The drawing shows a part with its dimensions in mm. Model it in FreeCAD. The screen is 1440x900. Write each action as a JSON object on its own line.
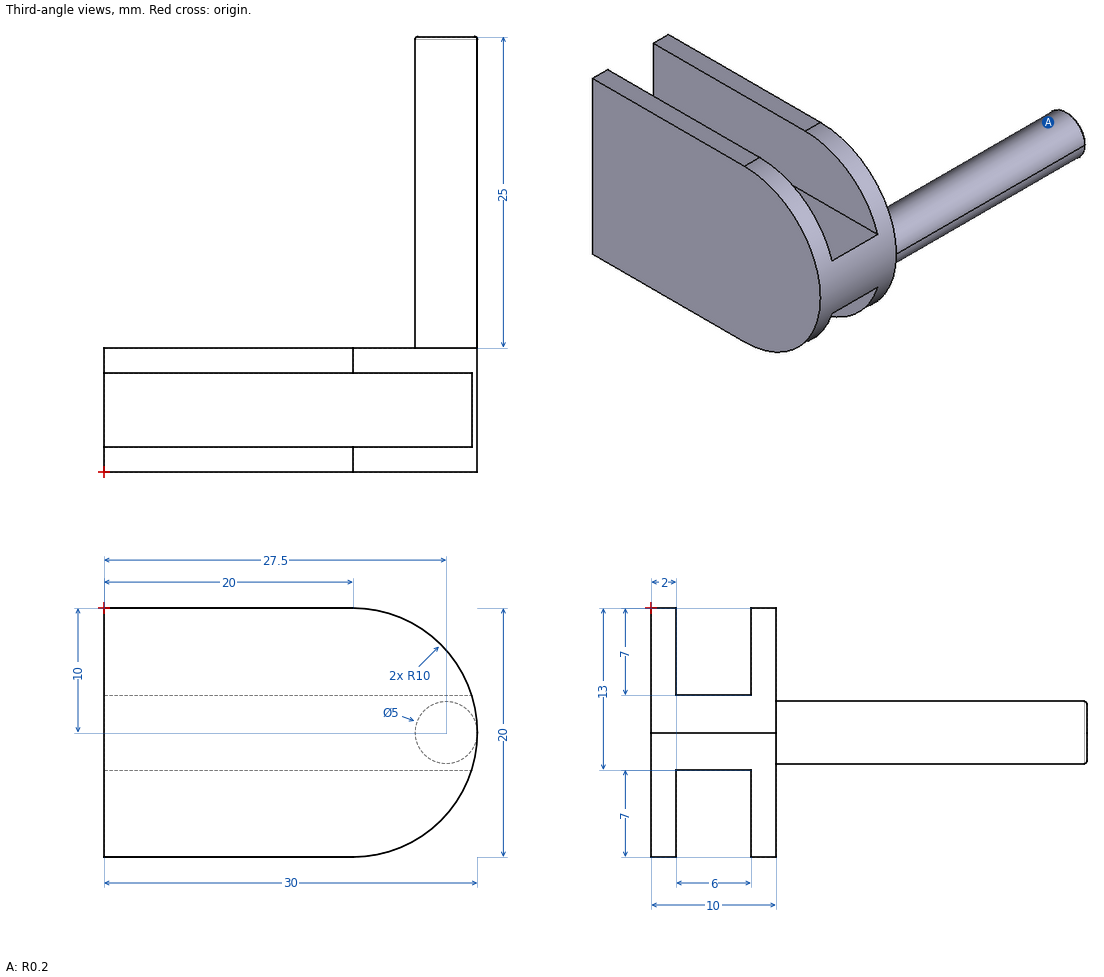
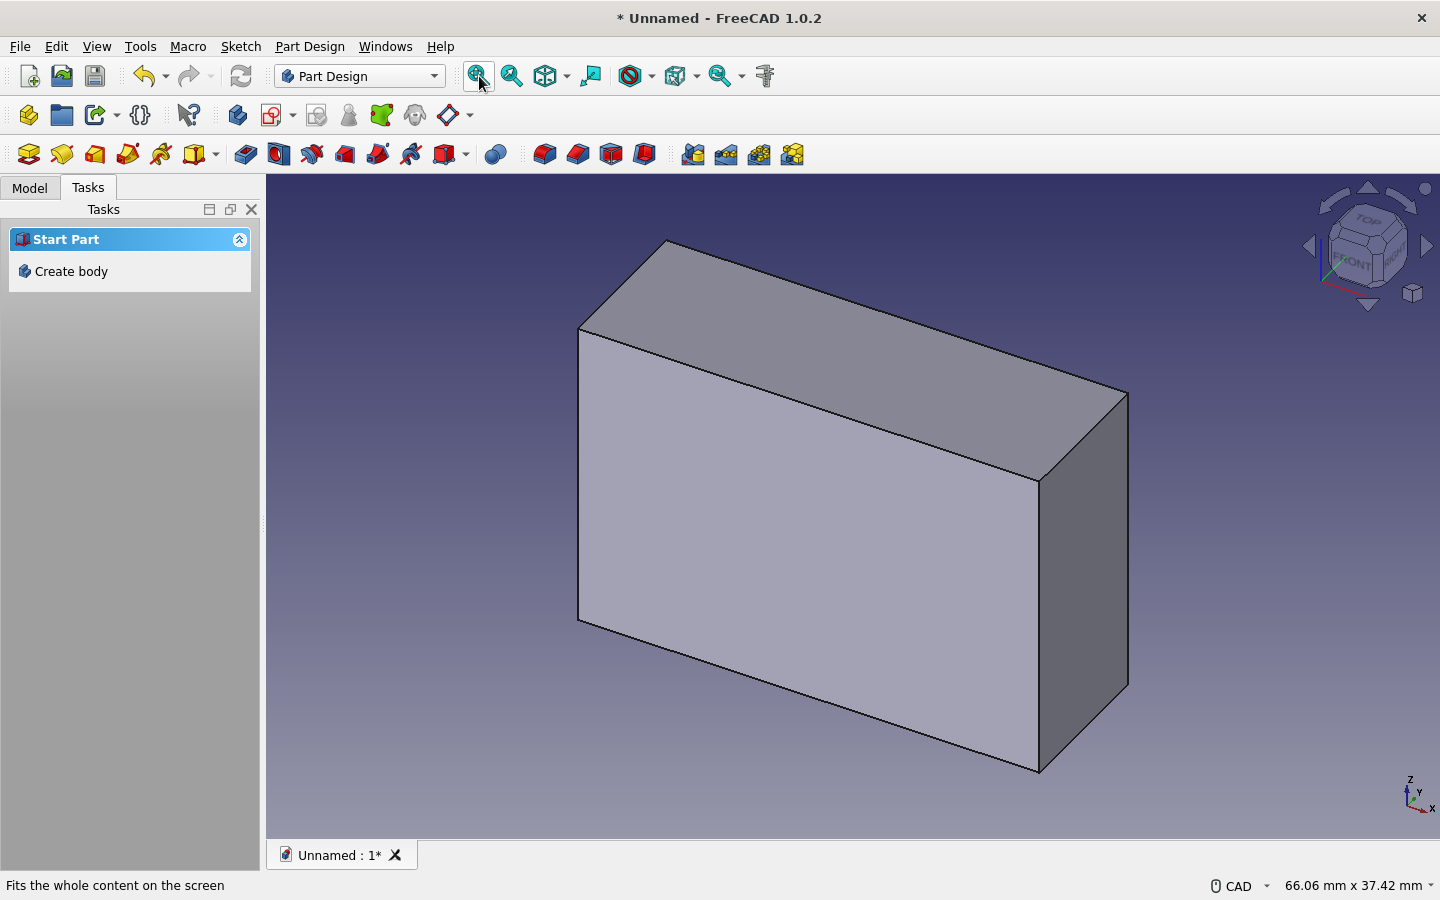
{"action": "key", "text": "6"}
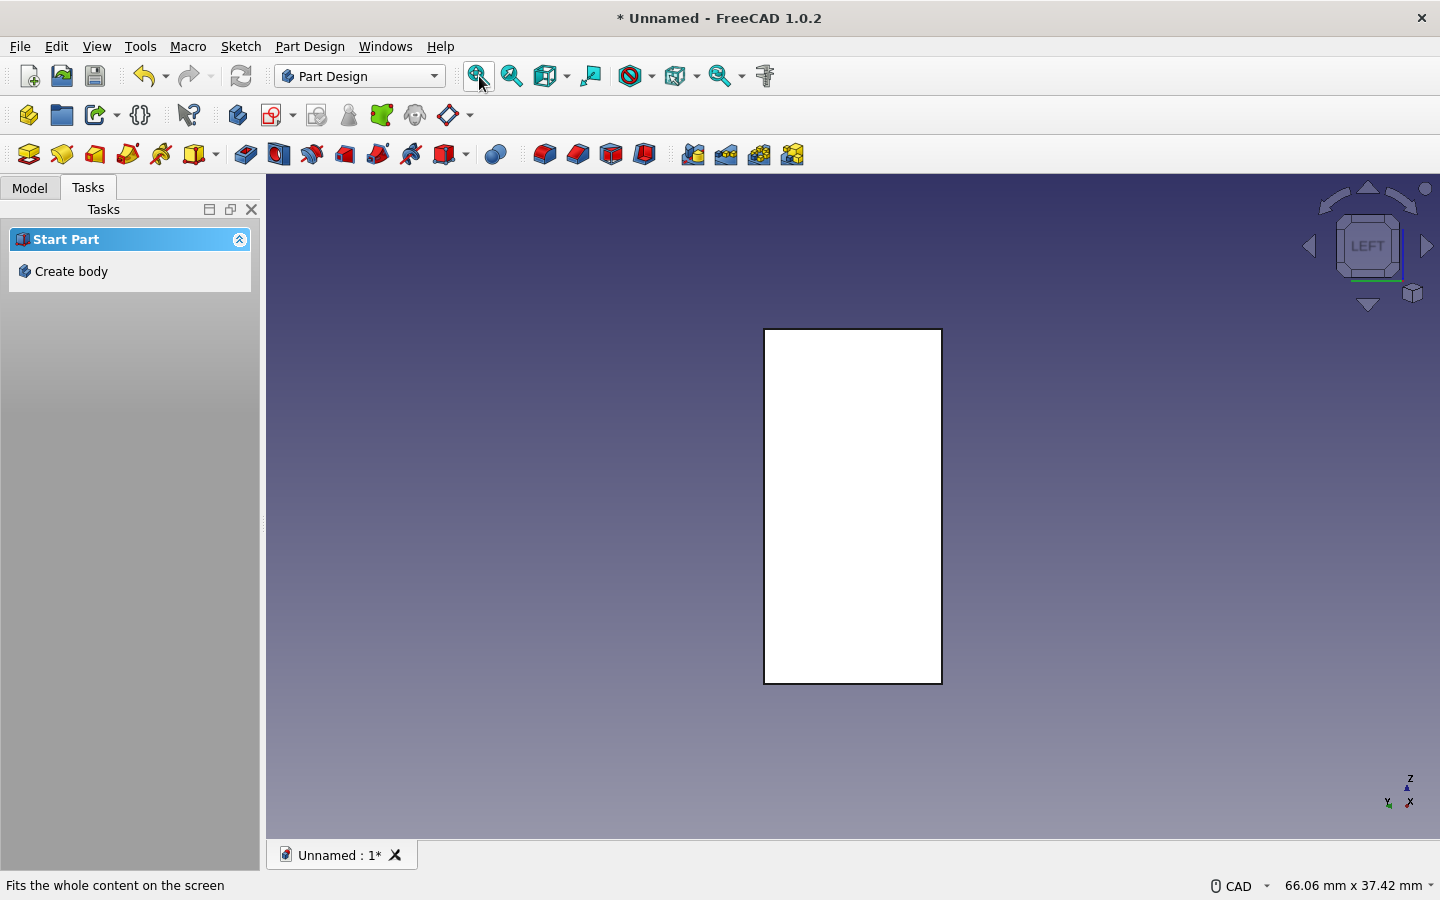
{"action": "left_click", "coordinate": [853, 455]}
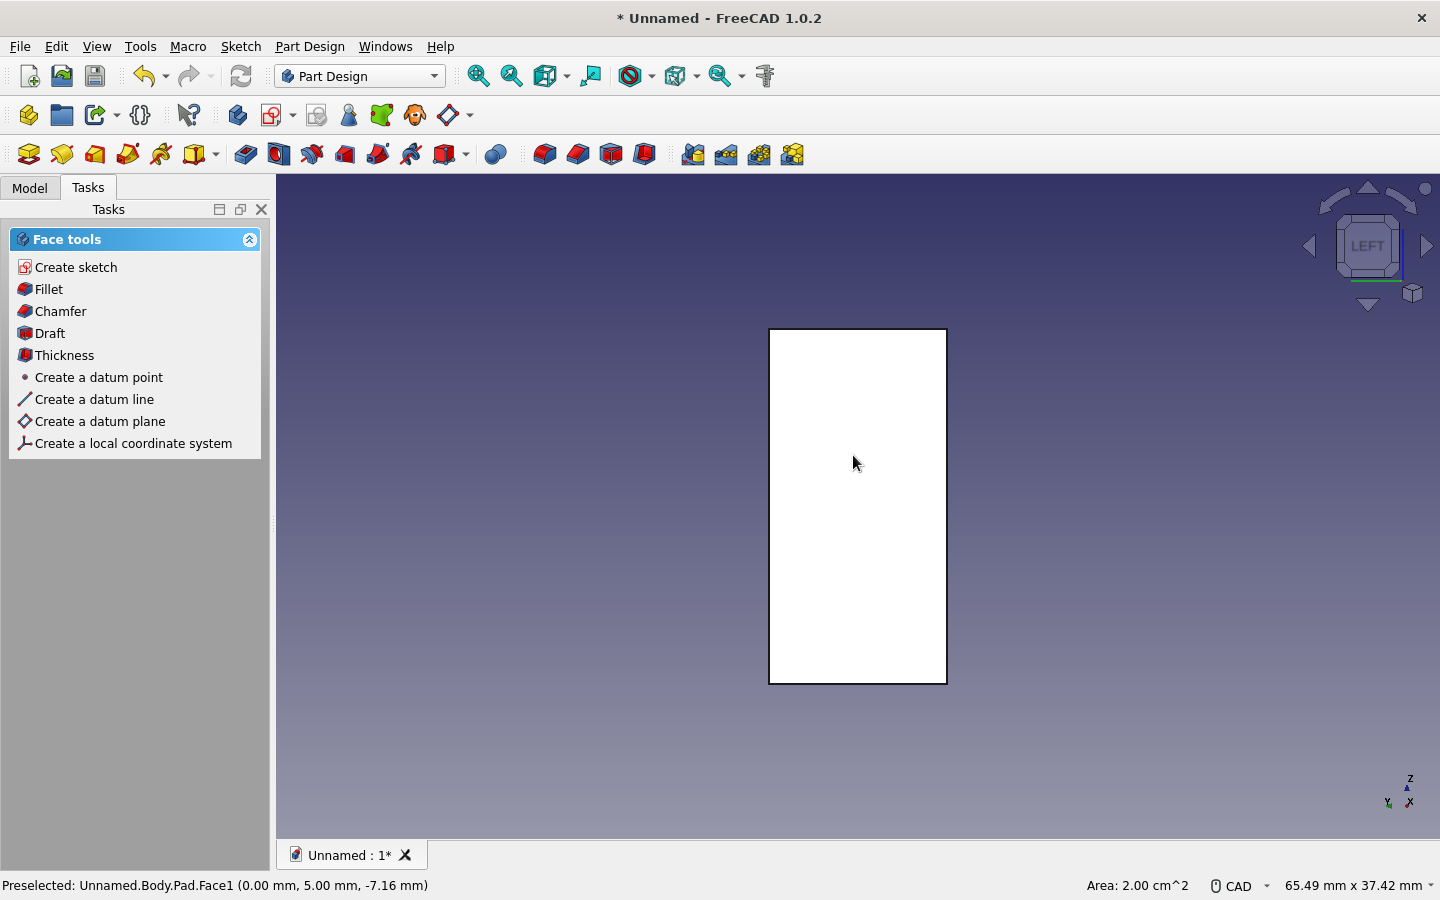
{"action": "left_click", "coordinate": [270, 116]}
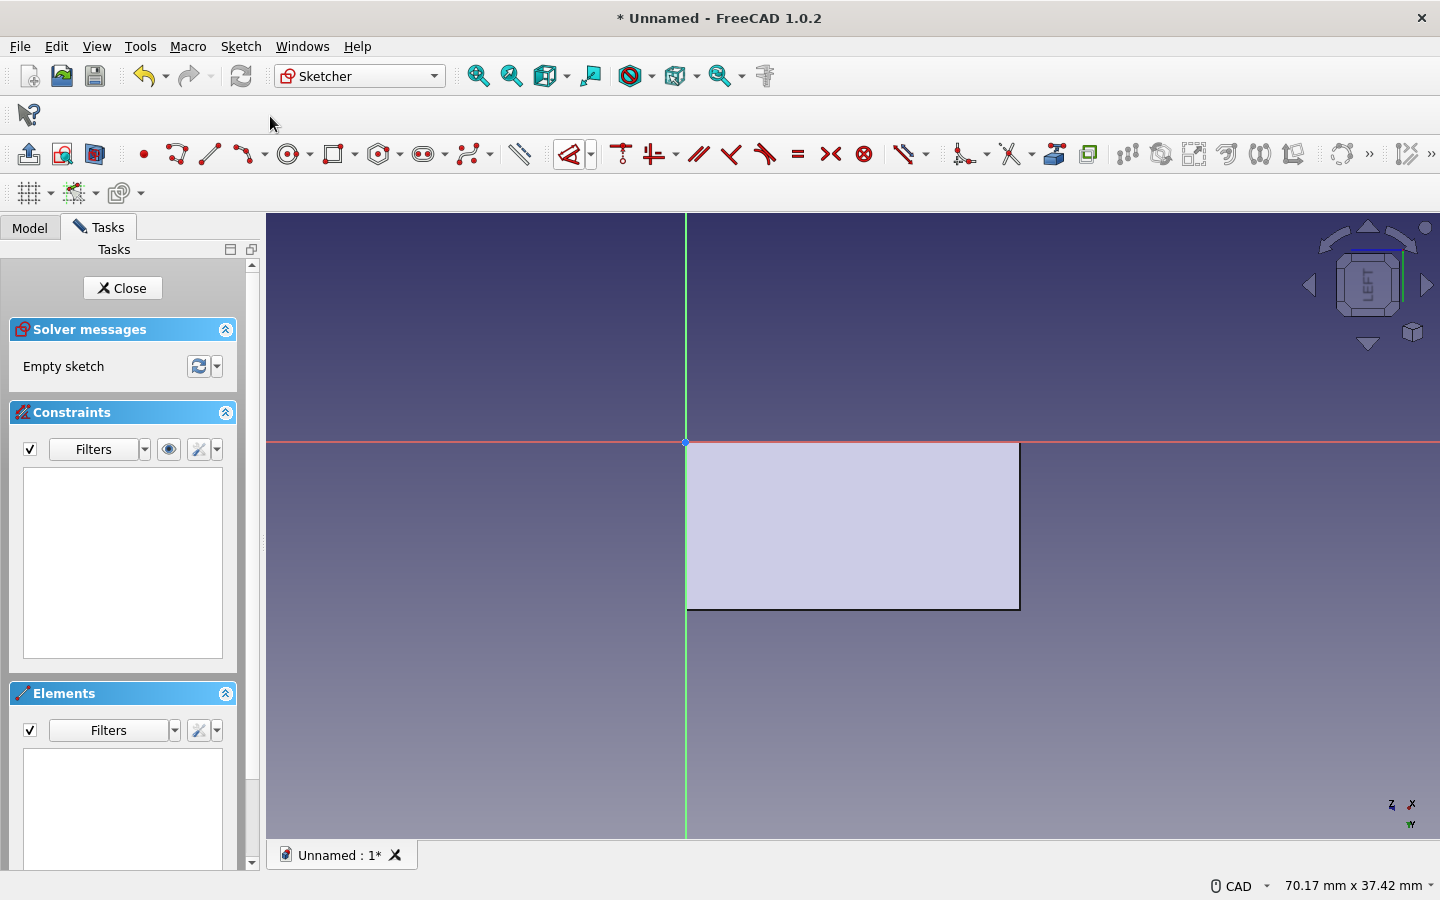
{"action": "scroll", "coordinate": [909, 496], "scroll_direction": "up", "scroll_amount": 4}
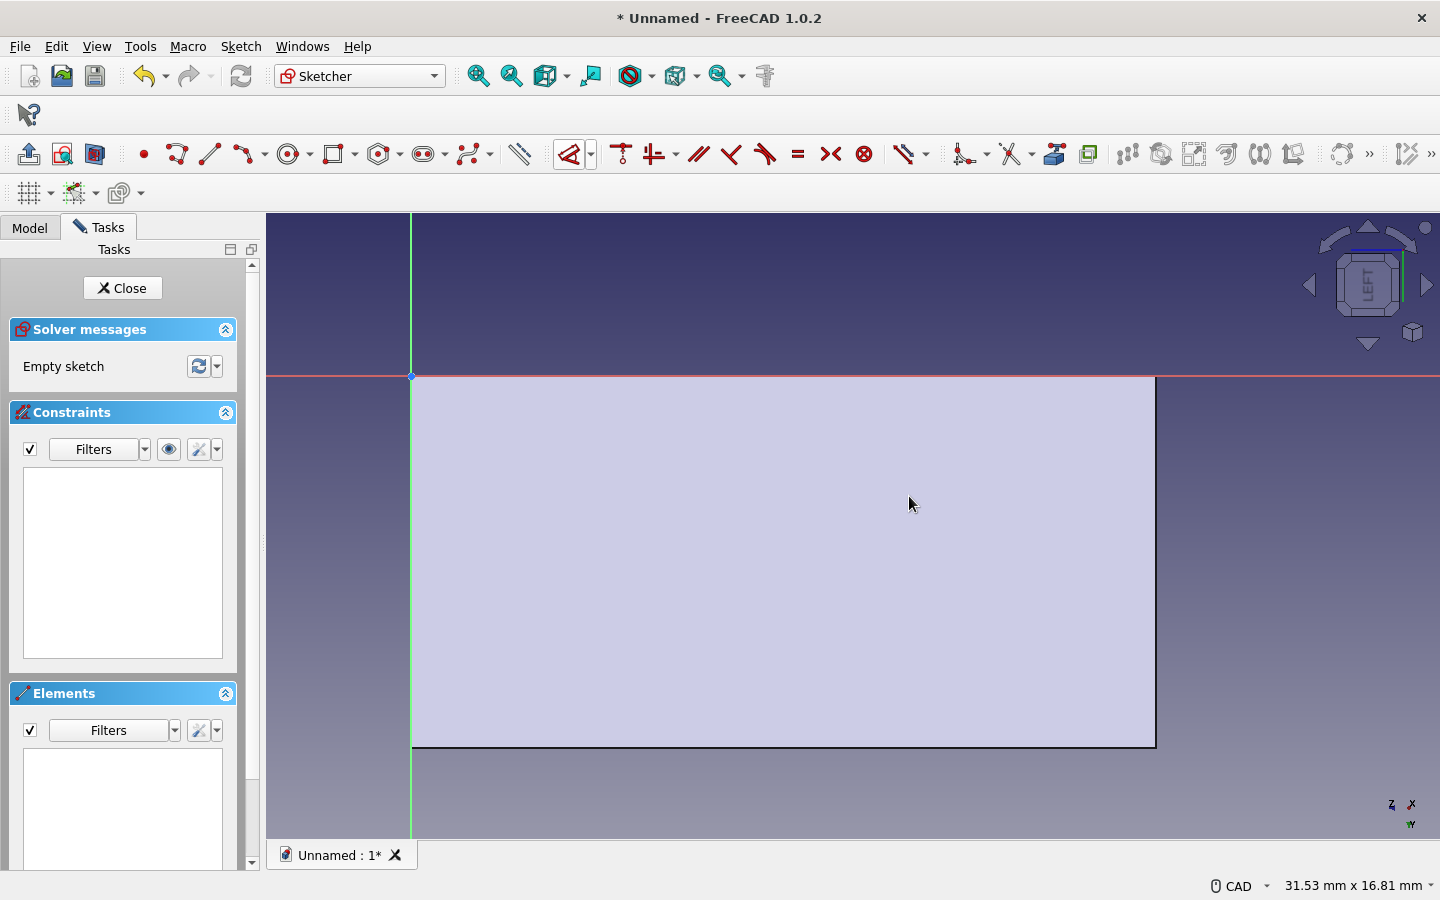
{"action": "left_click", "coordinate": [332, 154]}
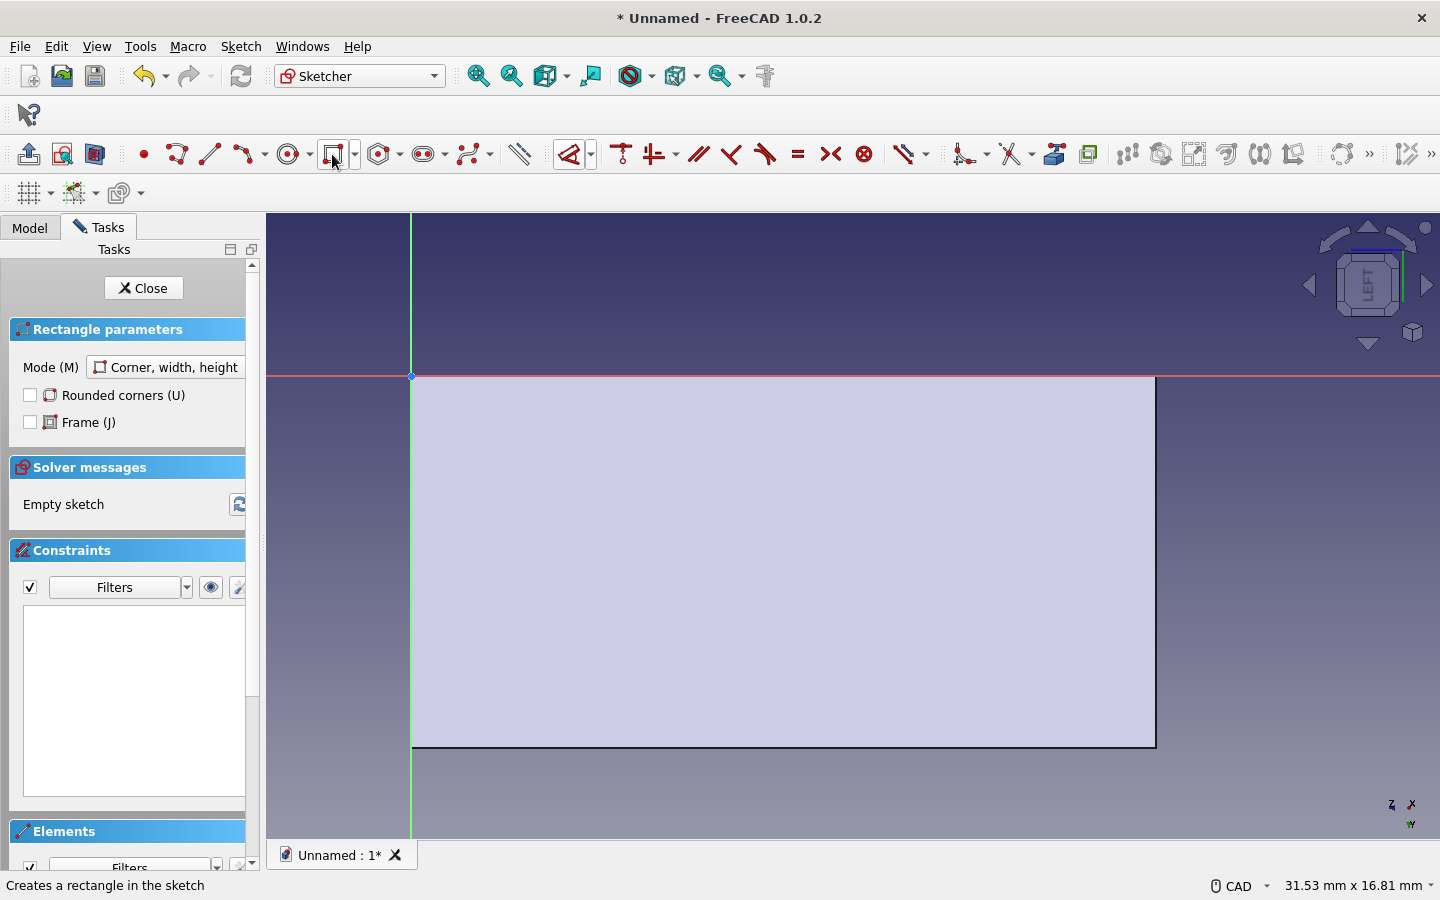
{"action": "left_click", "coordinate": [895, 451]}
{"action": "mouse_move", "coordinate": [1156, 674]}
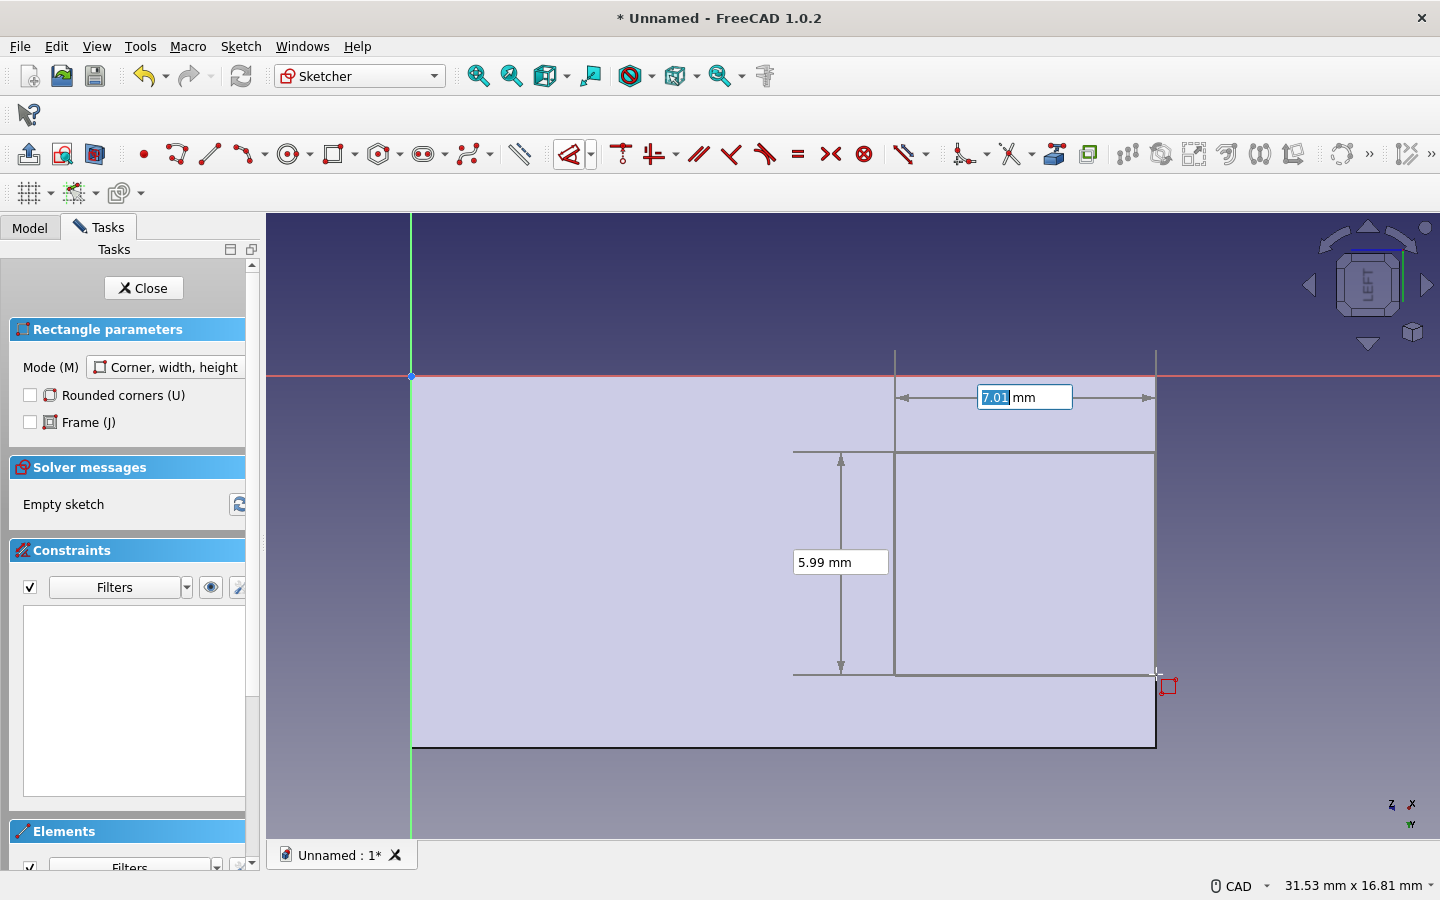
{"action": "type", "text": "7"}
{"action": "key", "text": "Tab"}
{"action": "type", "text": "6"}
{"action": "key", "text": "Return"}